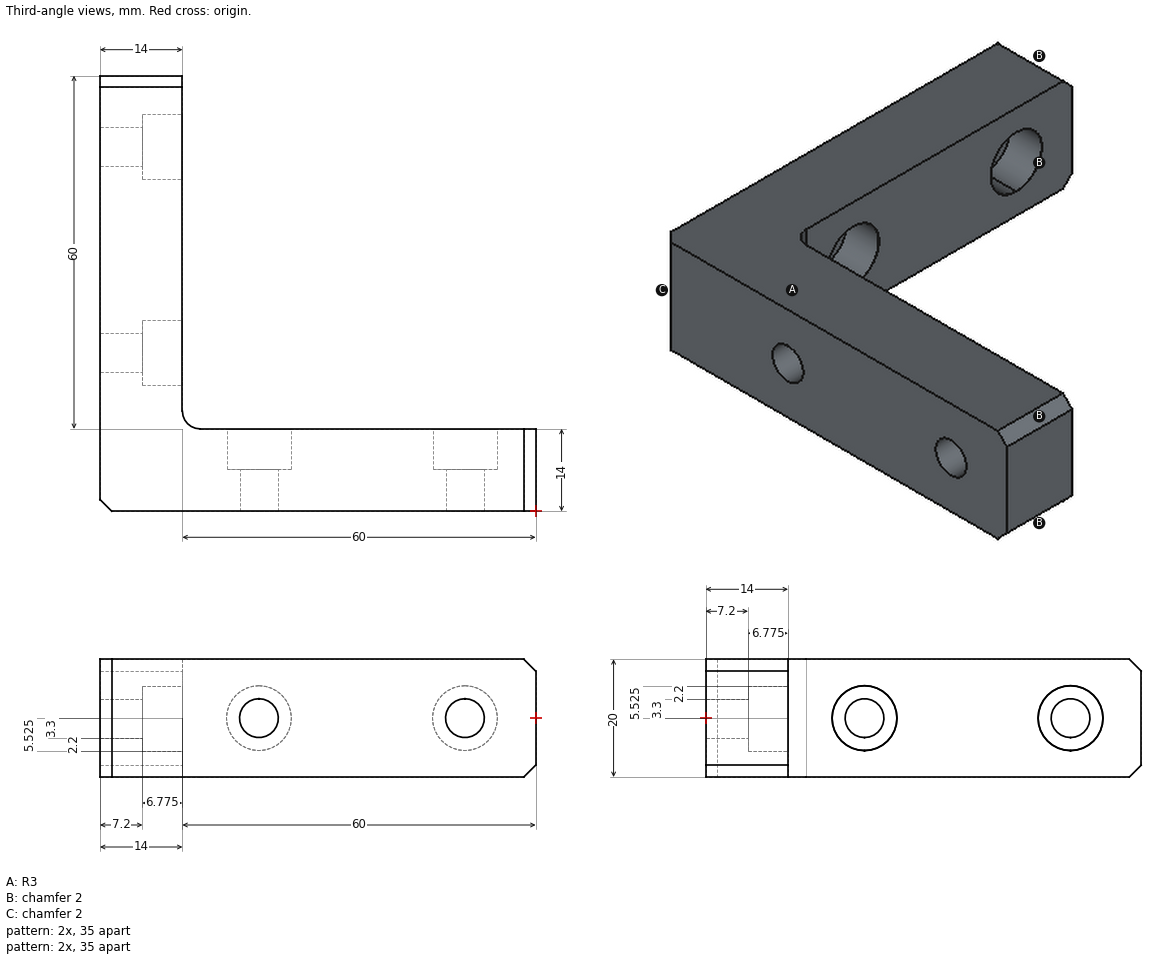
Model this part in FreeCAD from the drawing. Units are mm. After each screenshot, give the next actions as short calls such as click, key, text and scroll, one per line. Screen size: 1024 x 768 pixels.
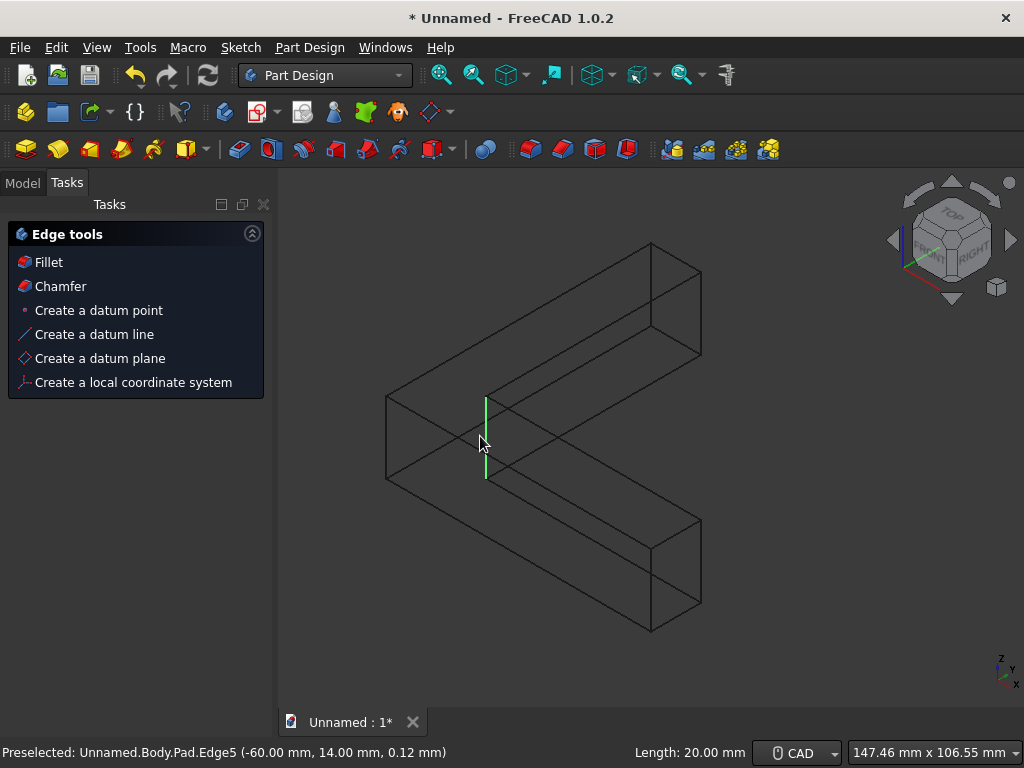
key(v)
key(1)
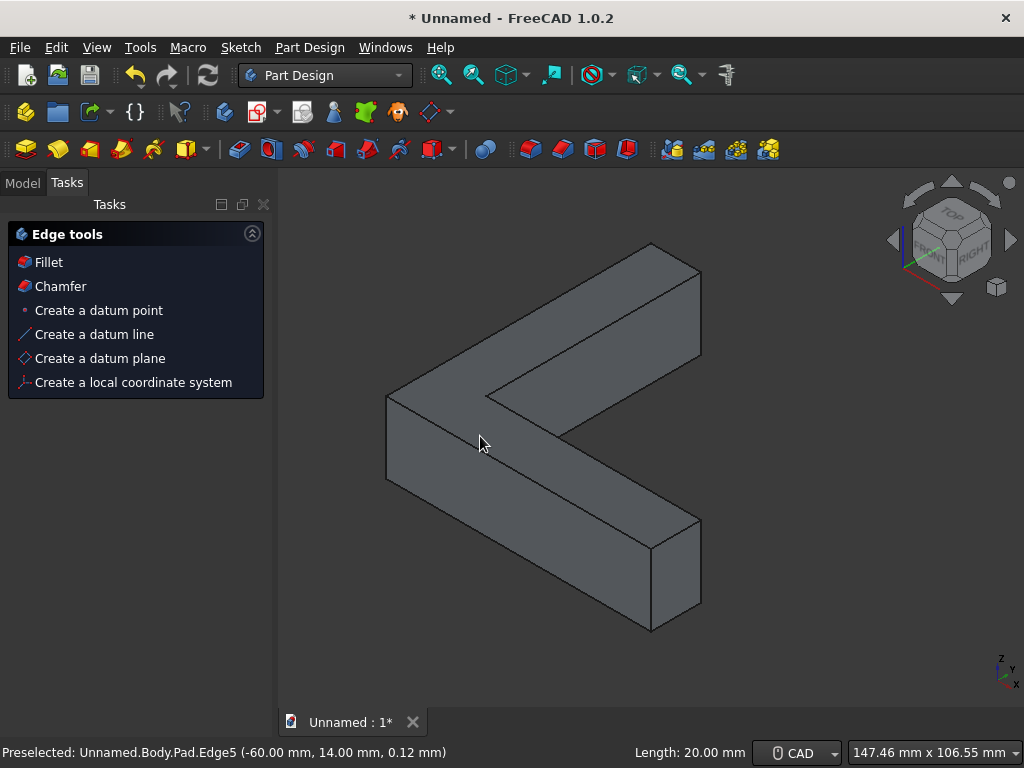
click(532, 150)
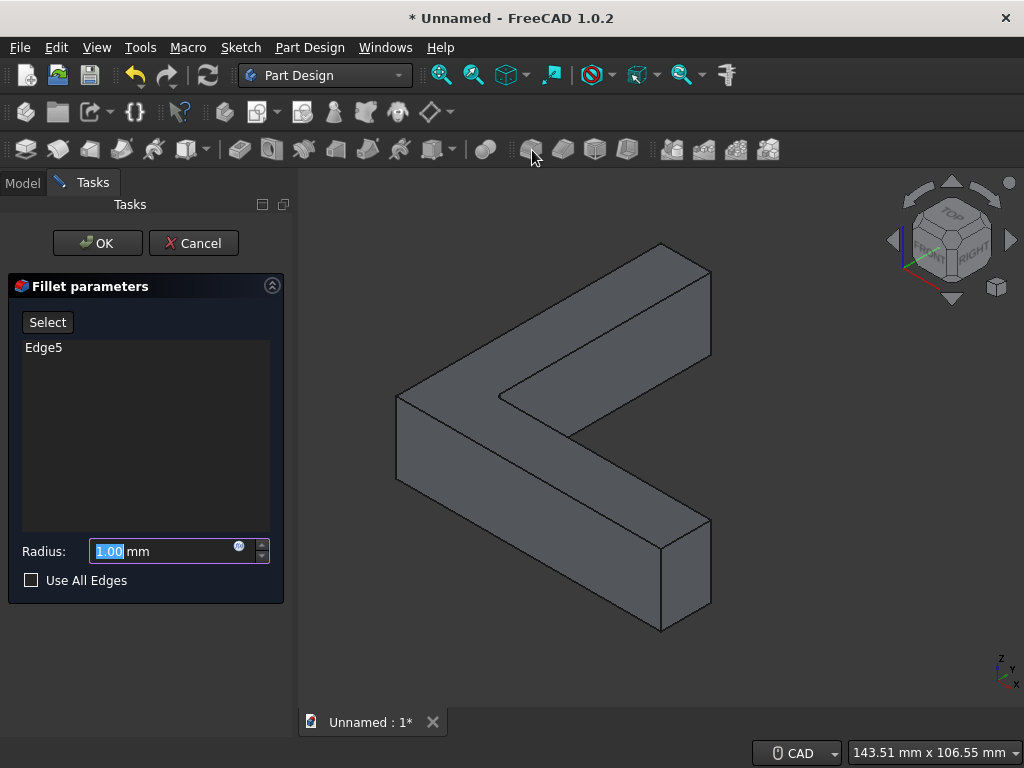
text(3)
key(Tab)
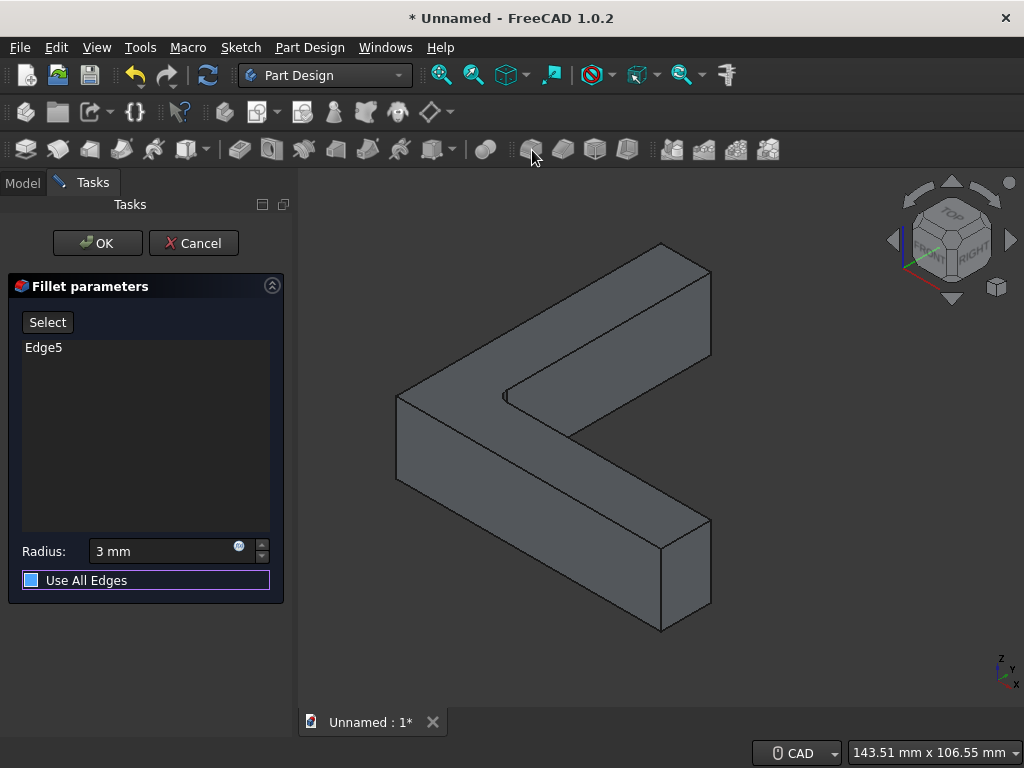
click(98, 243)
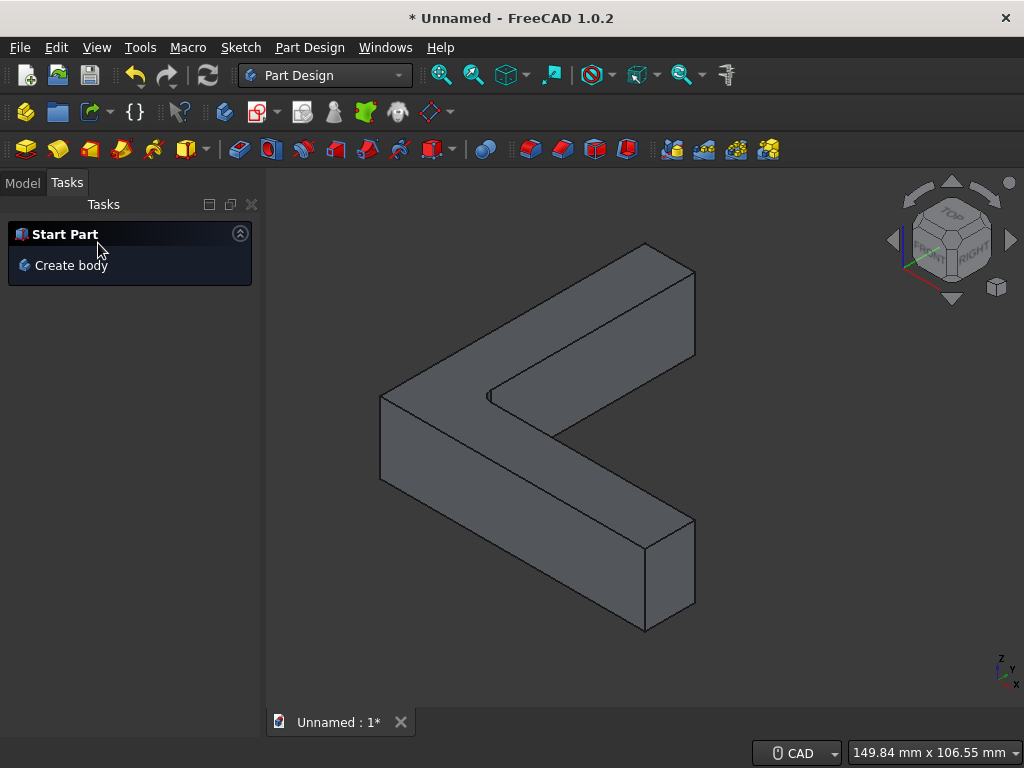
click(670, 534)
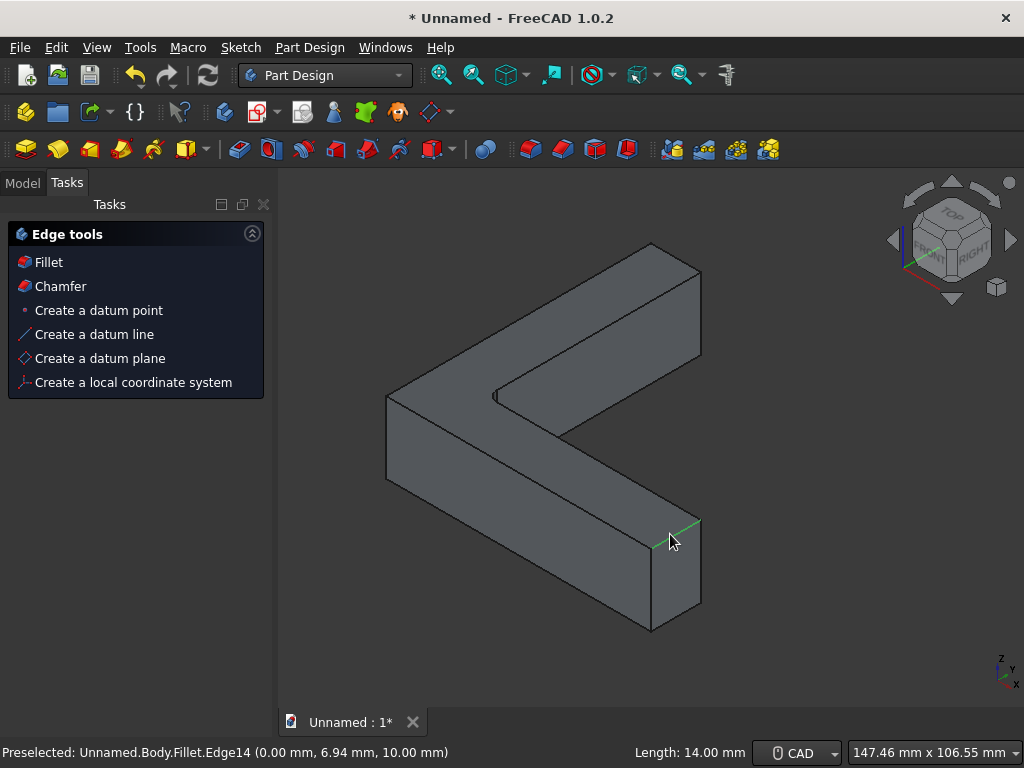
key(2)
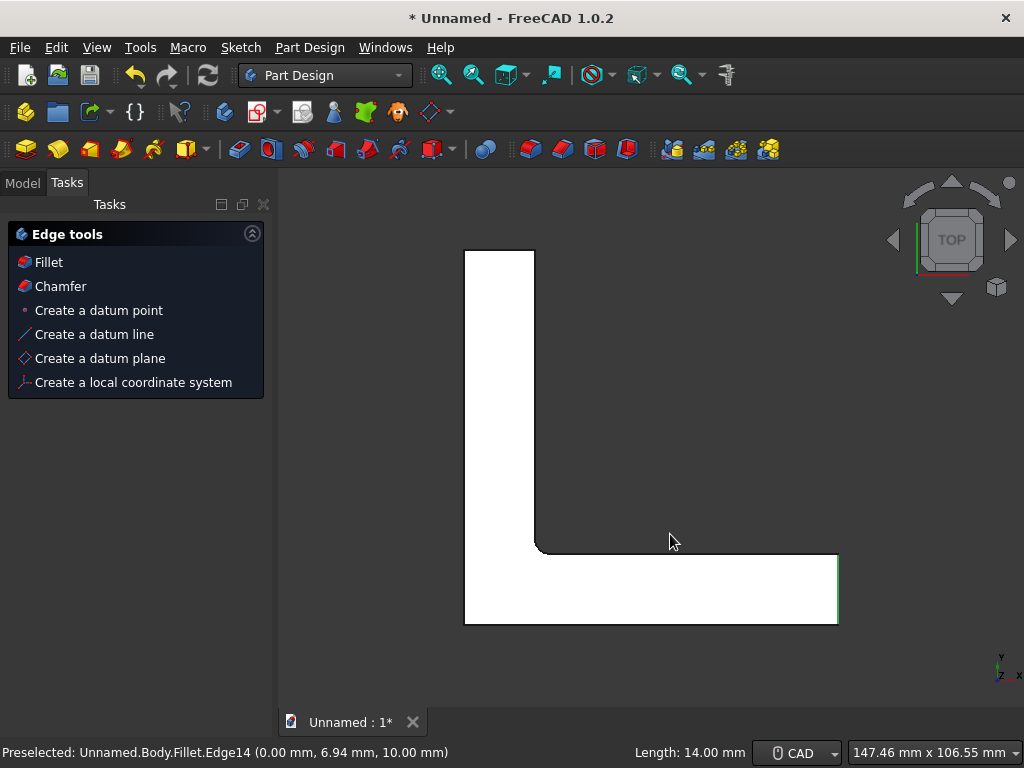
click(499, 249, ctrl)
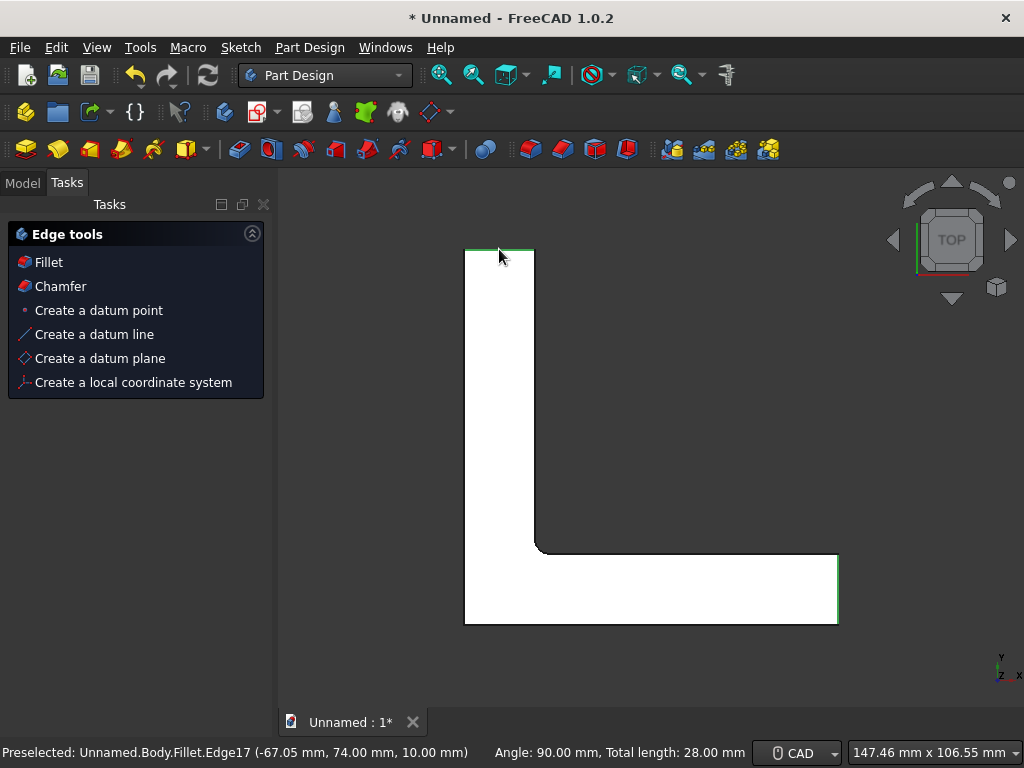
key(0)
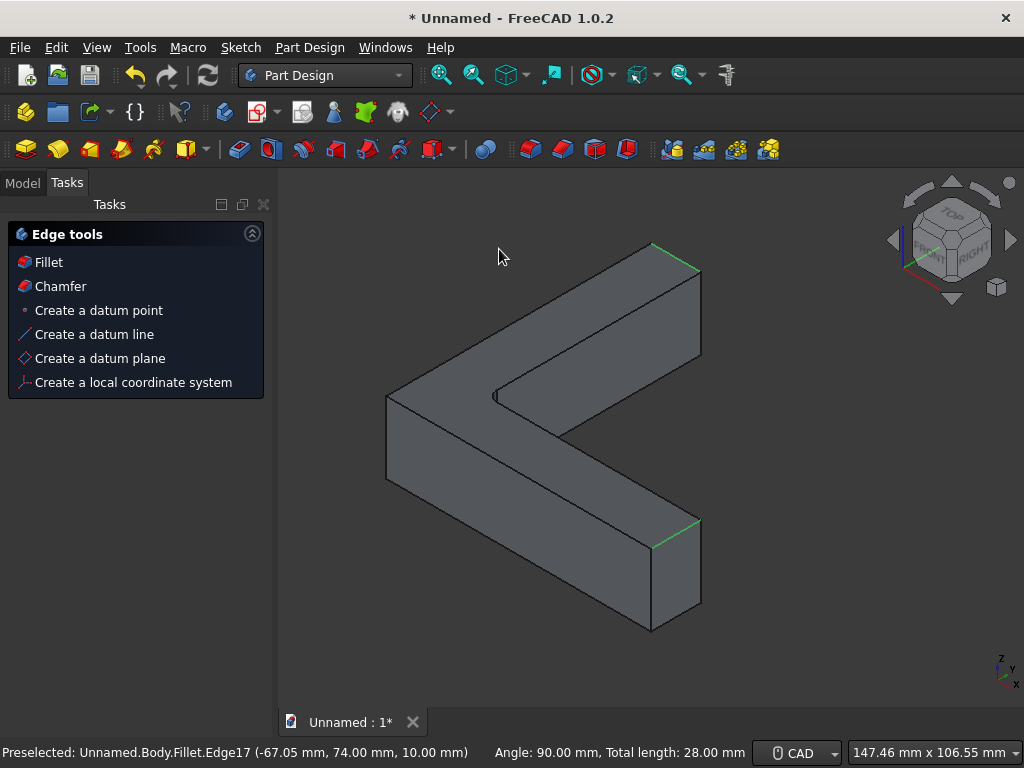
key(1)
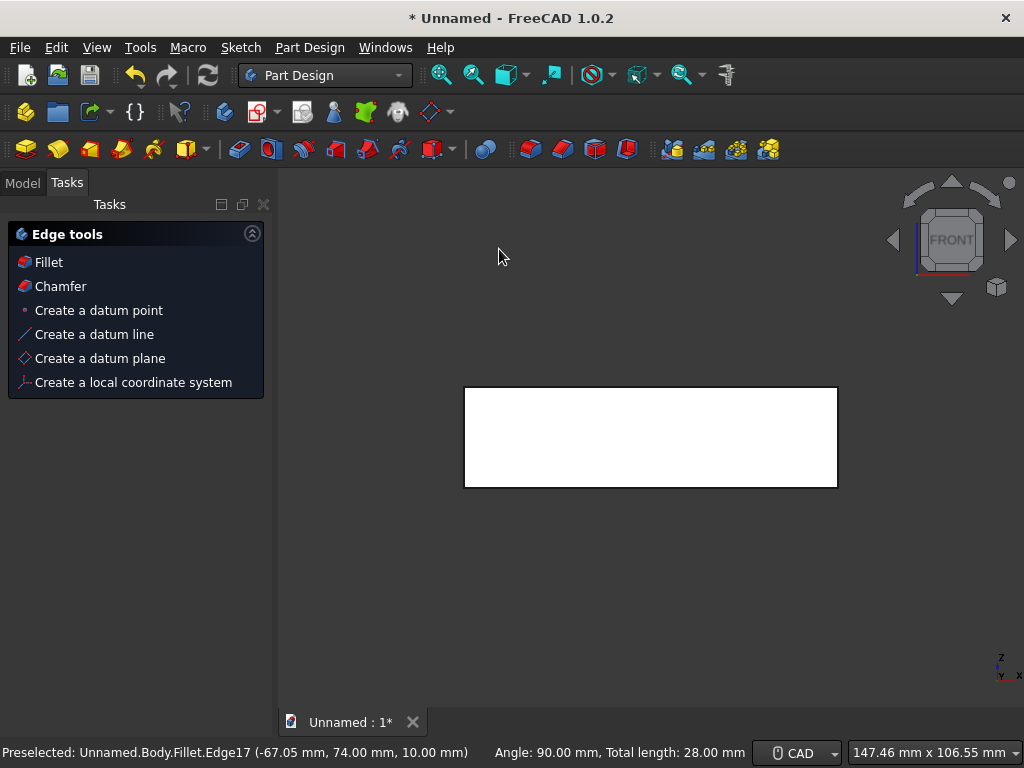
key(3)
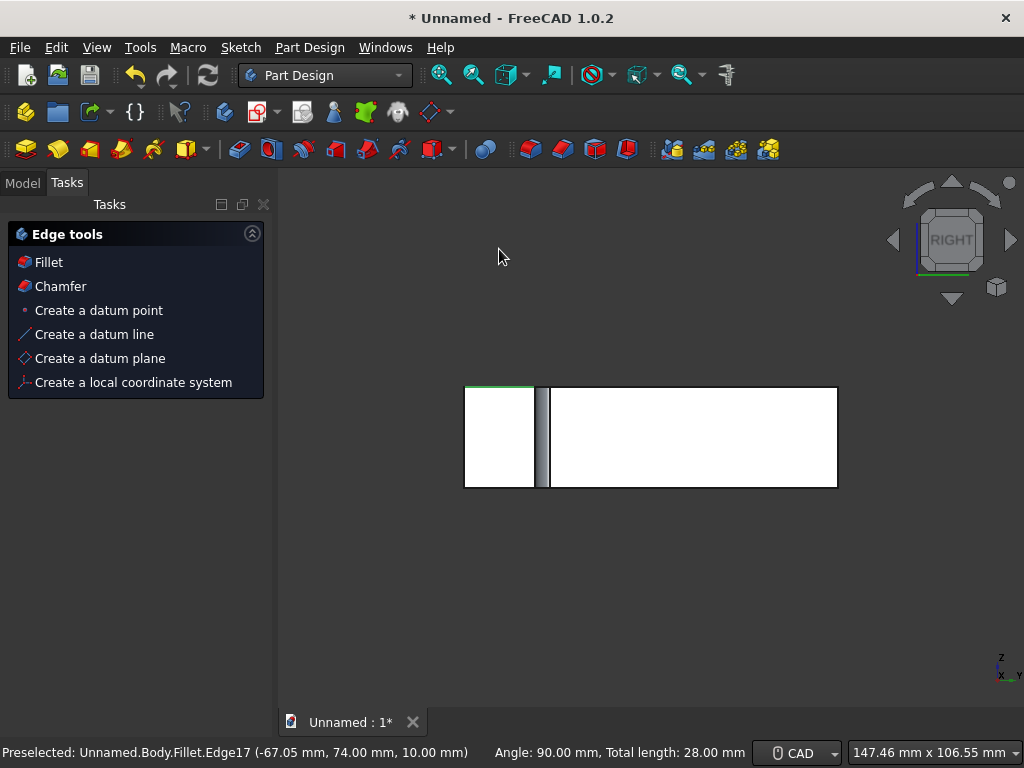
click(499, 487, ctrl)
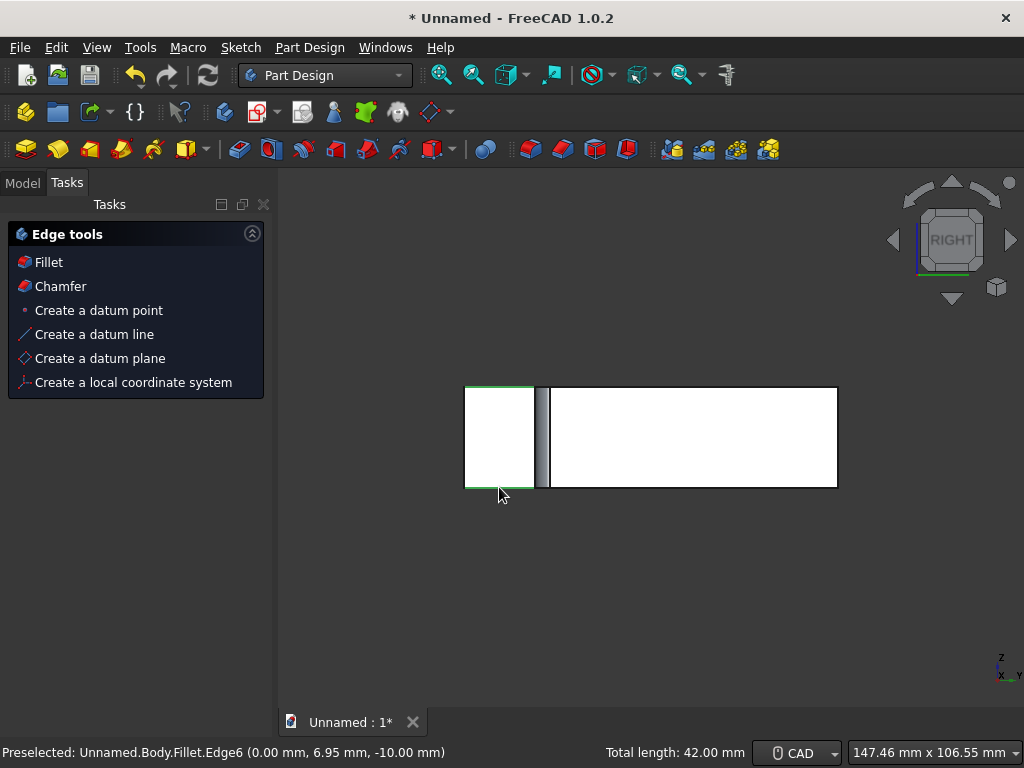
key(5)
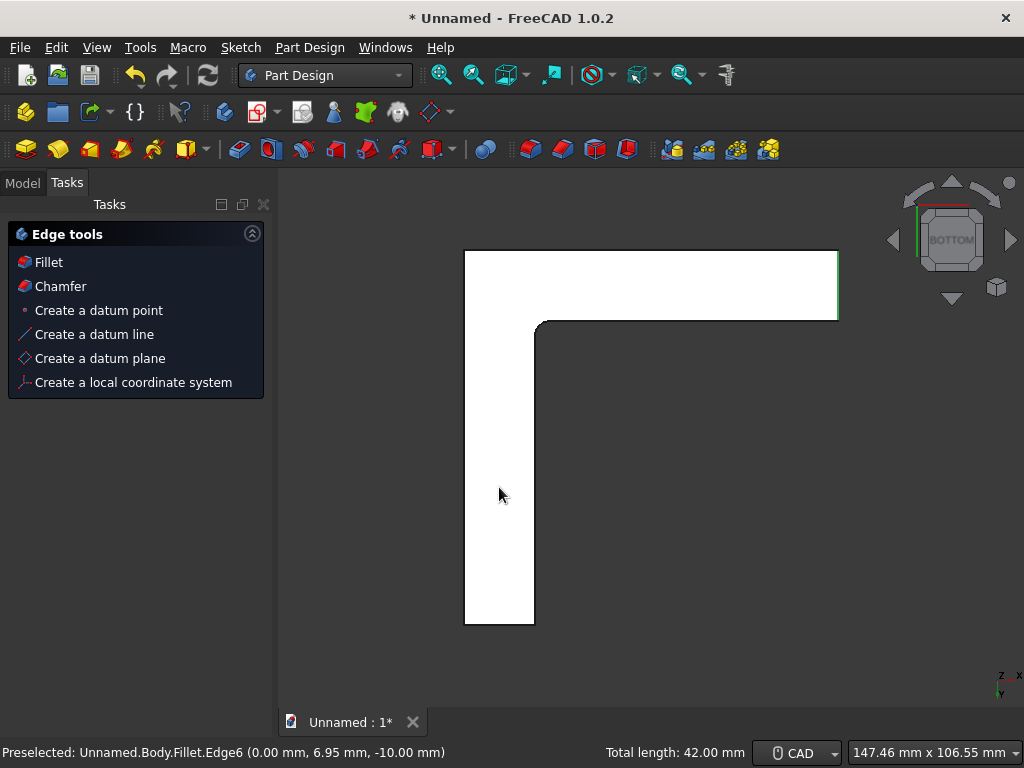
click(499, 624, ctrl)